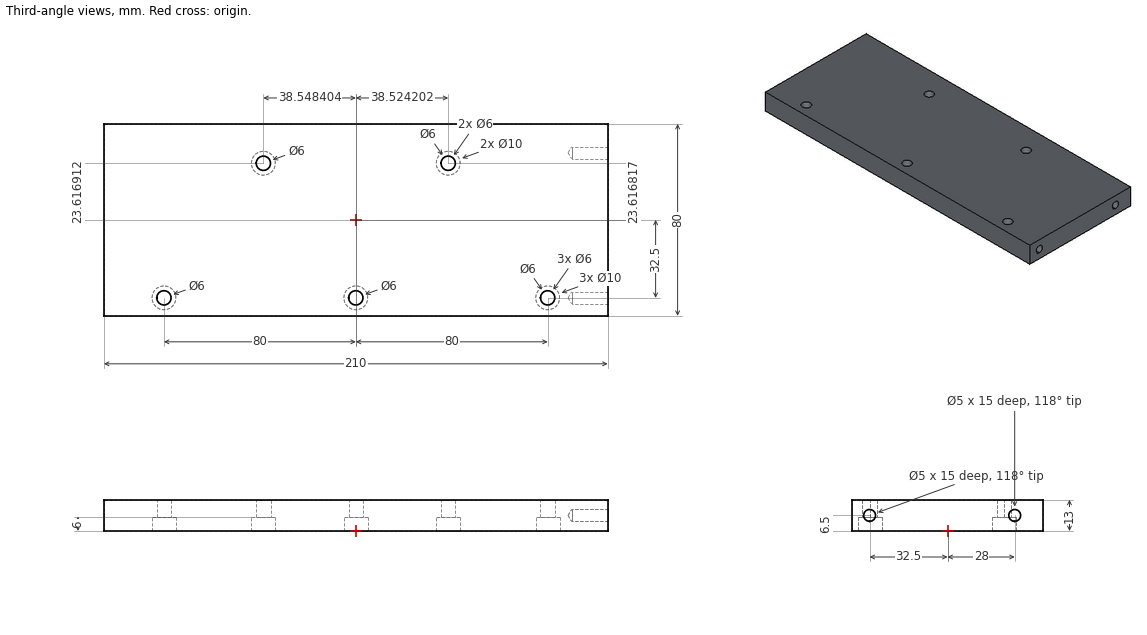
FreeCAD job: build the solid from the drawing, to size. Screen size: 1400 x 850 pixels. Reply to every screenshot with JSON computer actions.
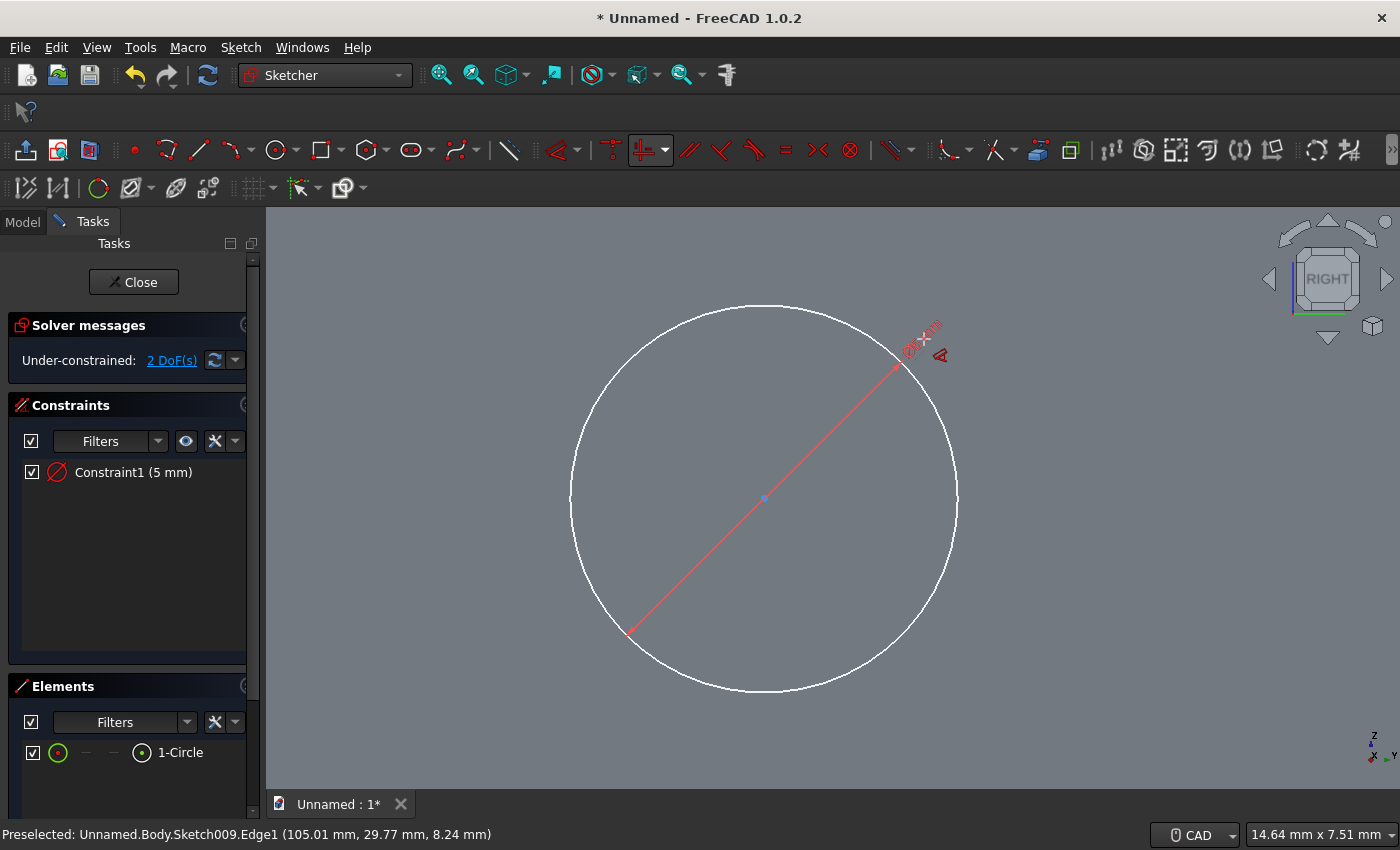
{"action": "left_click", "coordinate": [764, 499]}
{"action": "left_click", "coordinate": [529, 465]}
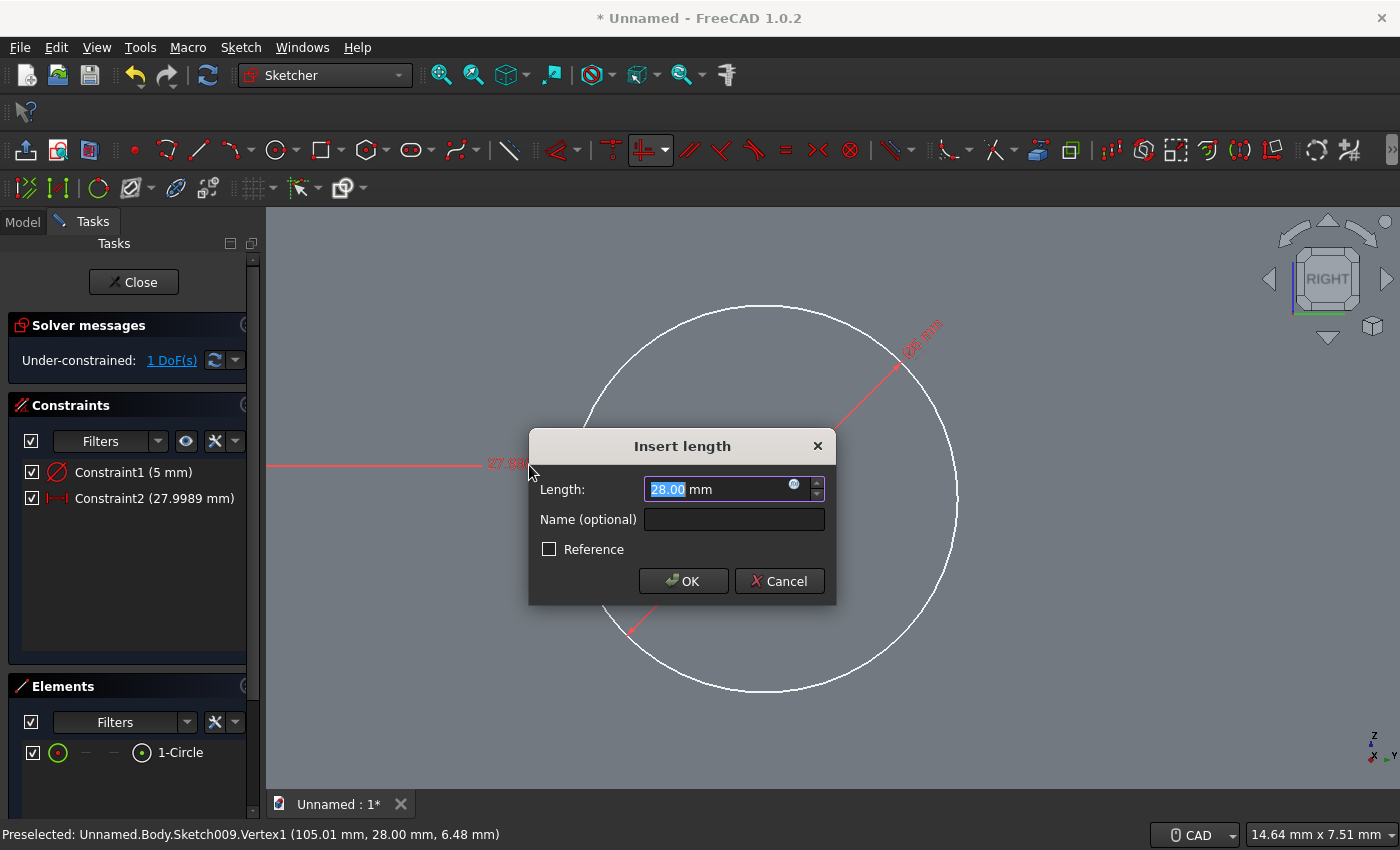
{"action": "type", "text": "28"}
{"action": "key", "text": "Return"}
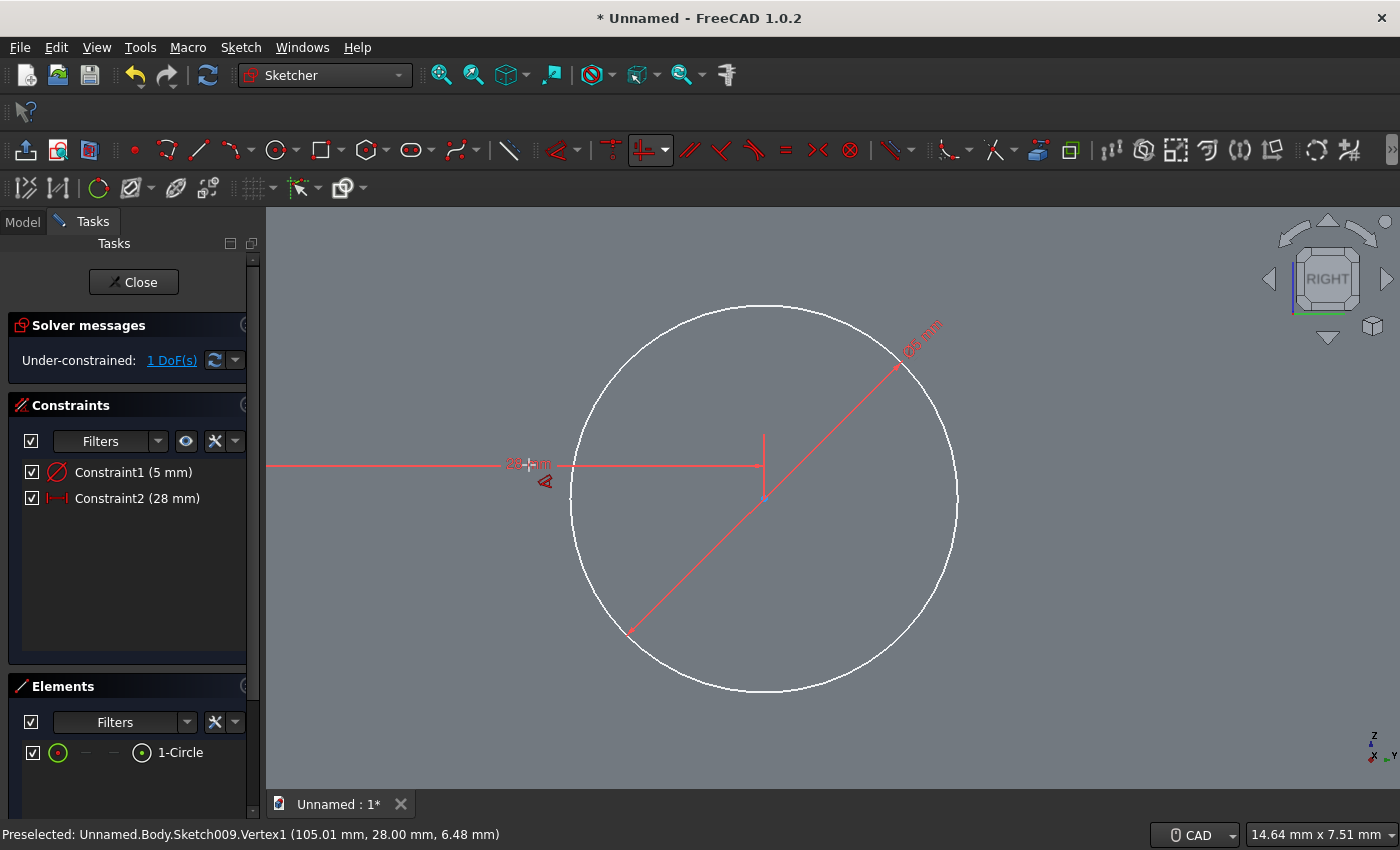
{"action": "left_click", "coordinate": [764, 499]}
{"action": "left_click", "coordinate": [798, 630]}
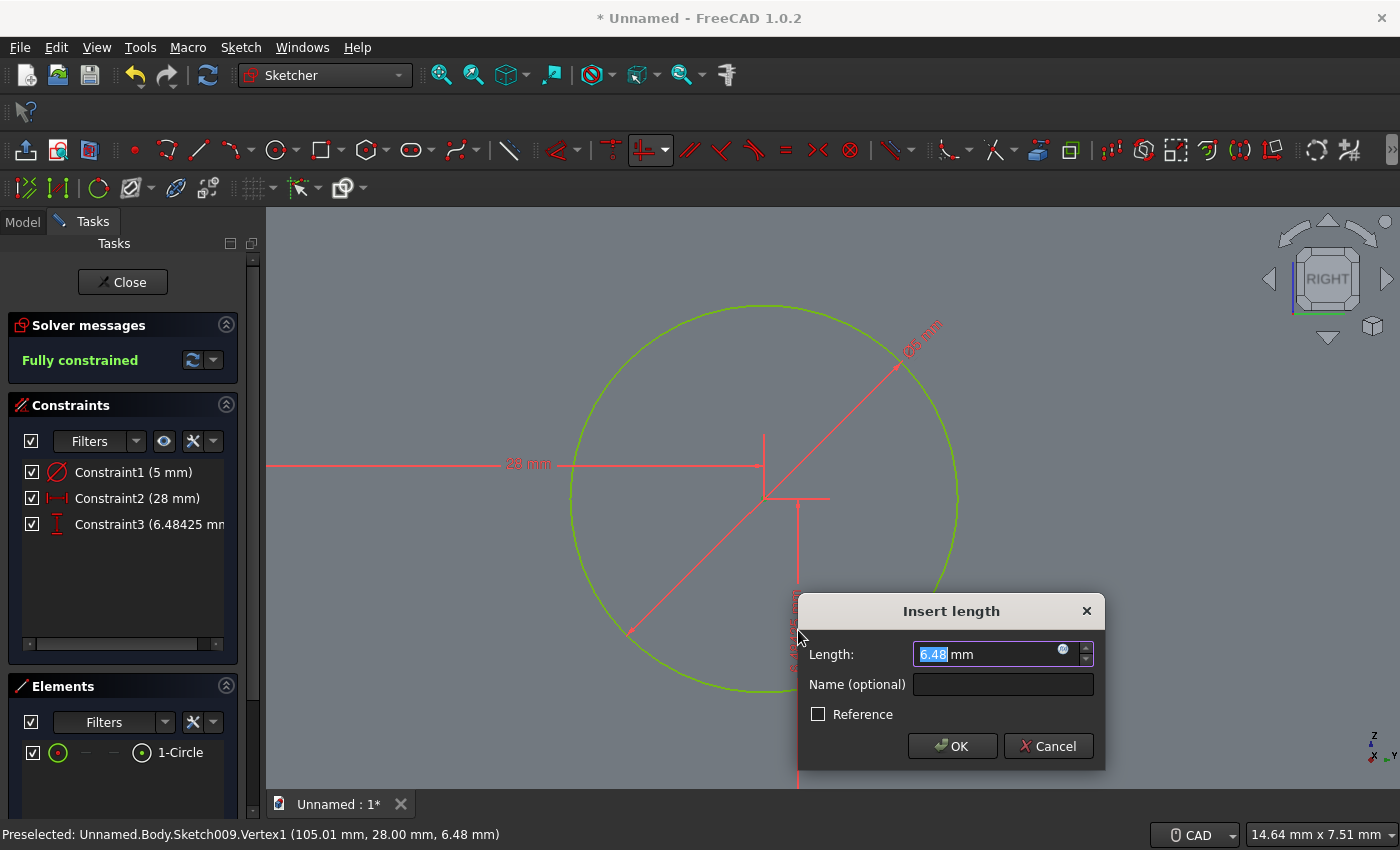
{"action": "type", "text": "6.5"}
{"action": "key", "text": "Return"}
{"action": "key", "text": "Escape"}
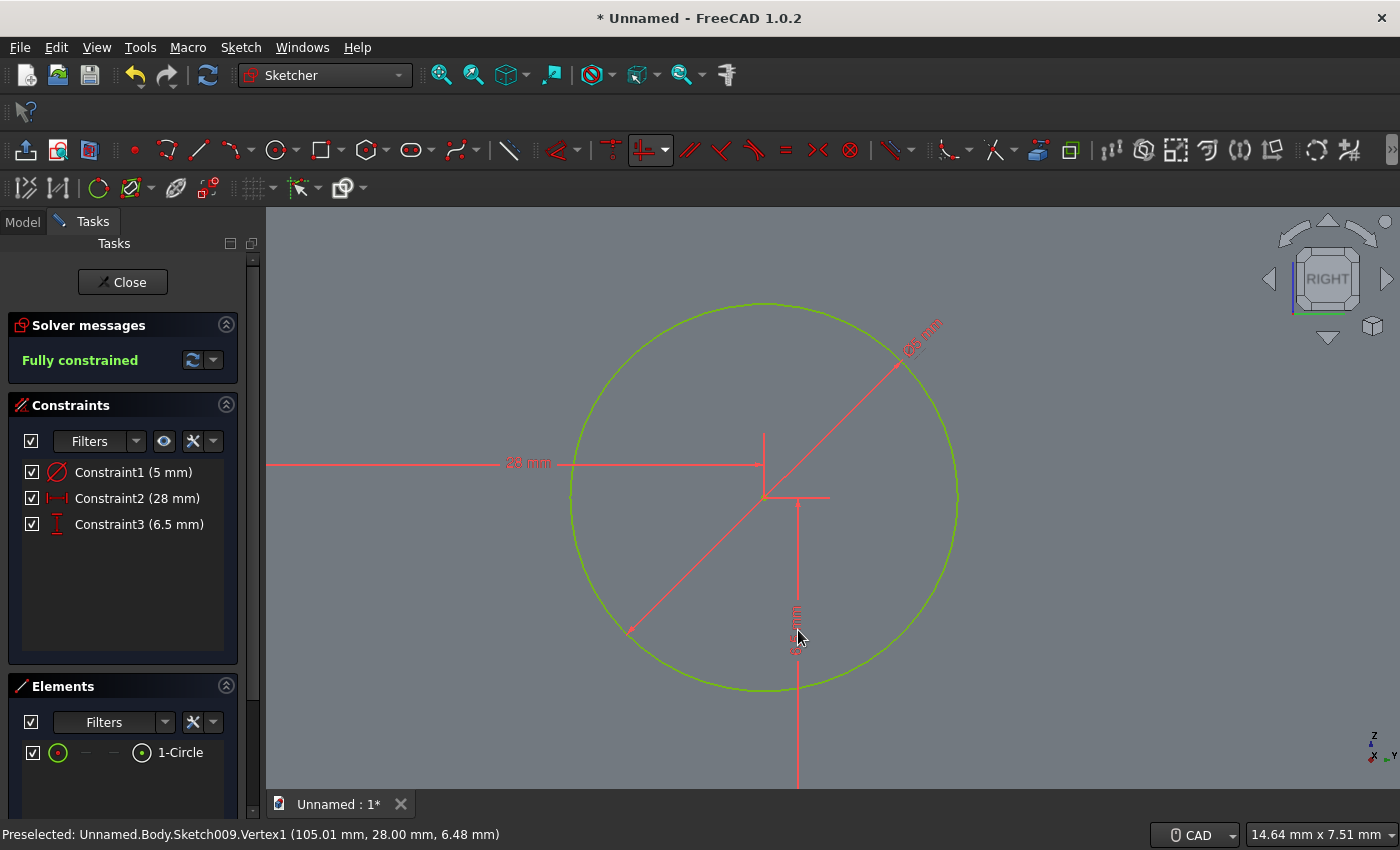
{"action": "left_click", "coordinate": [123, 282]}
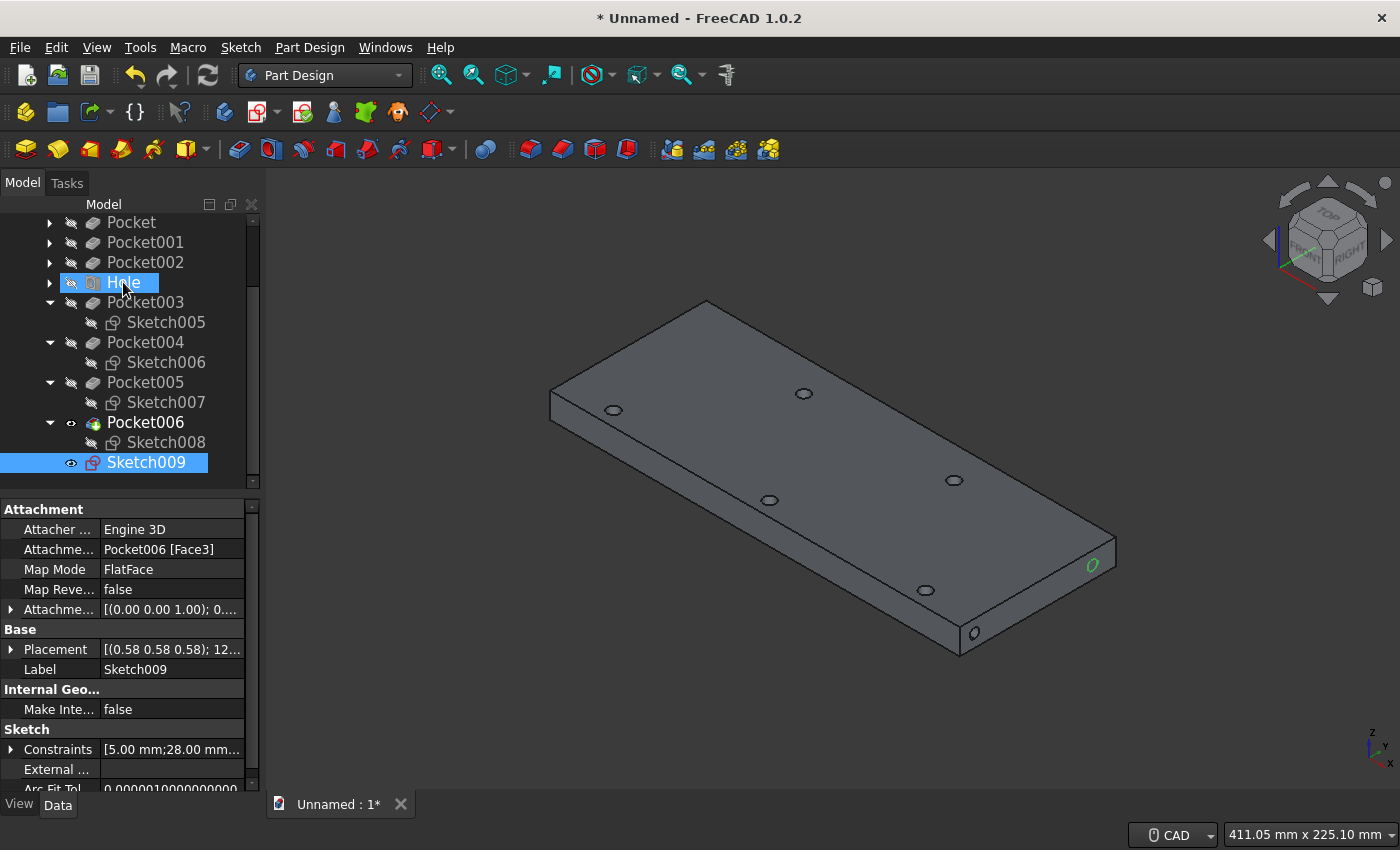
{"action": "left_click", "coordinate": [272, 150]}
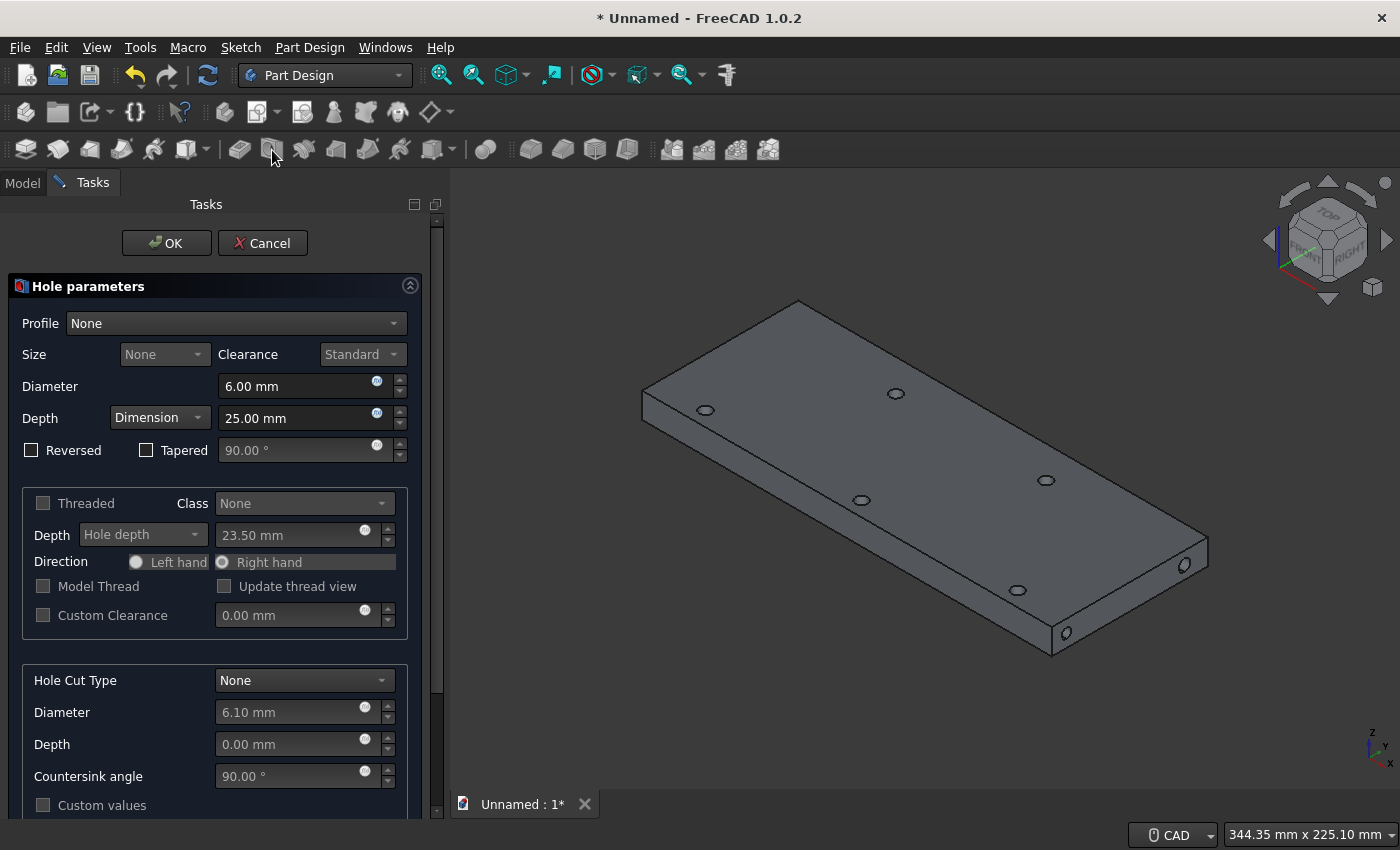
{"action": "triple_click", "coordinate": [305, 386]}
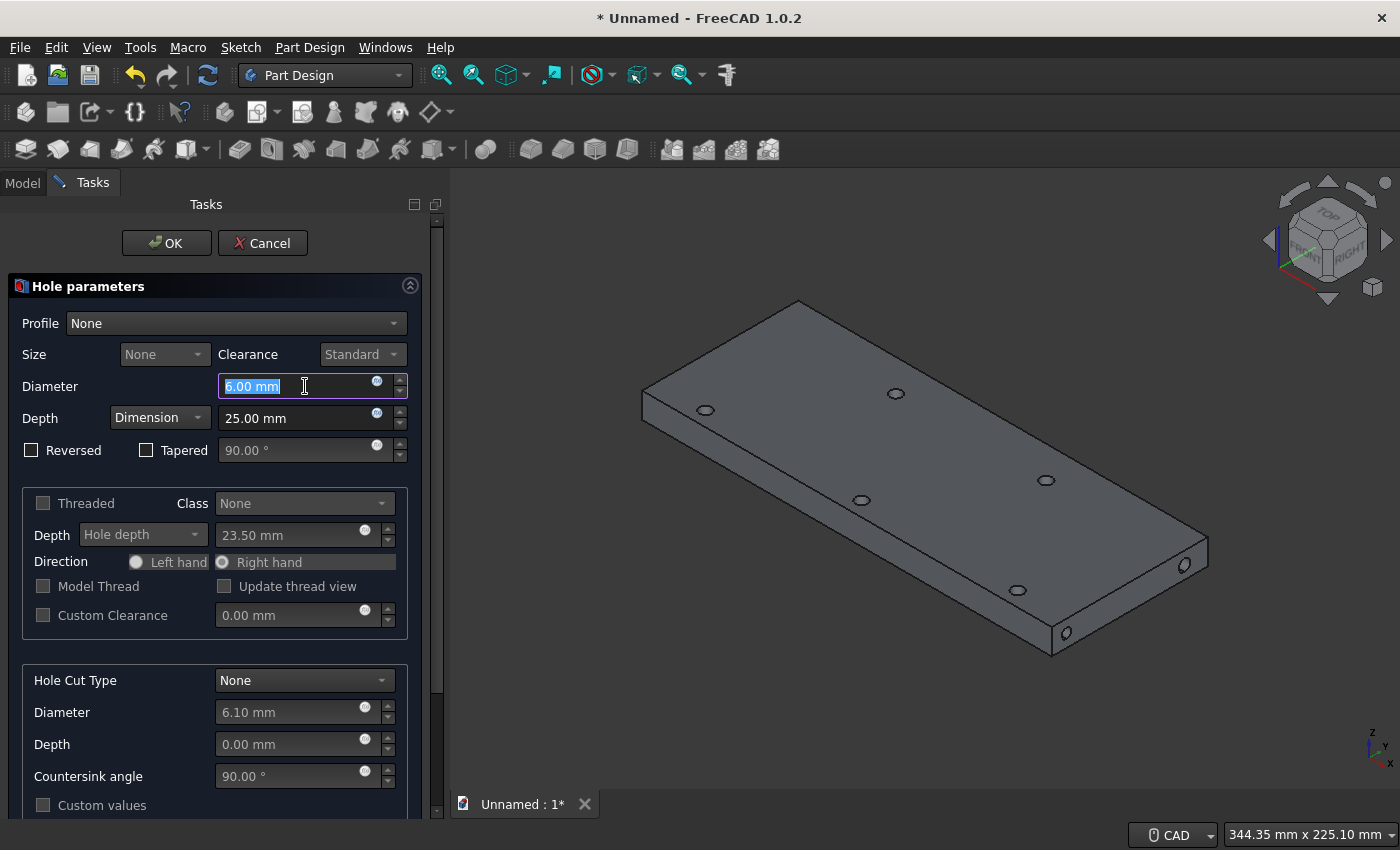
{"action": "type", "text": "5"}
{"action": "key", "text": "Tab"}